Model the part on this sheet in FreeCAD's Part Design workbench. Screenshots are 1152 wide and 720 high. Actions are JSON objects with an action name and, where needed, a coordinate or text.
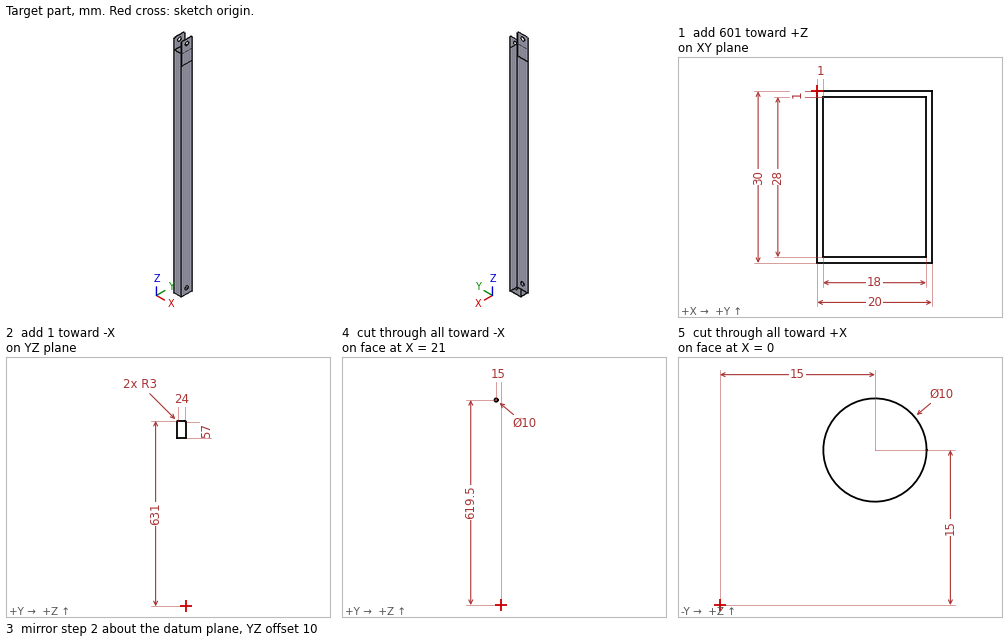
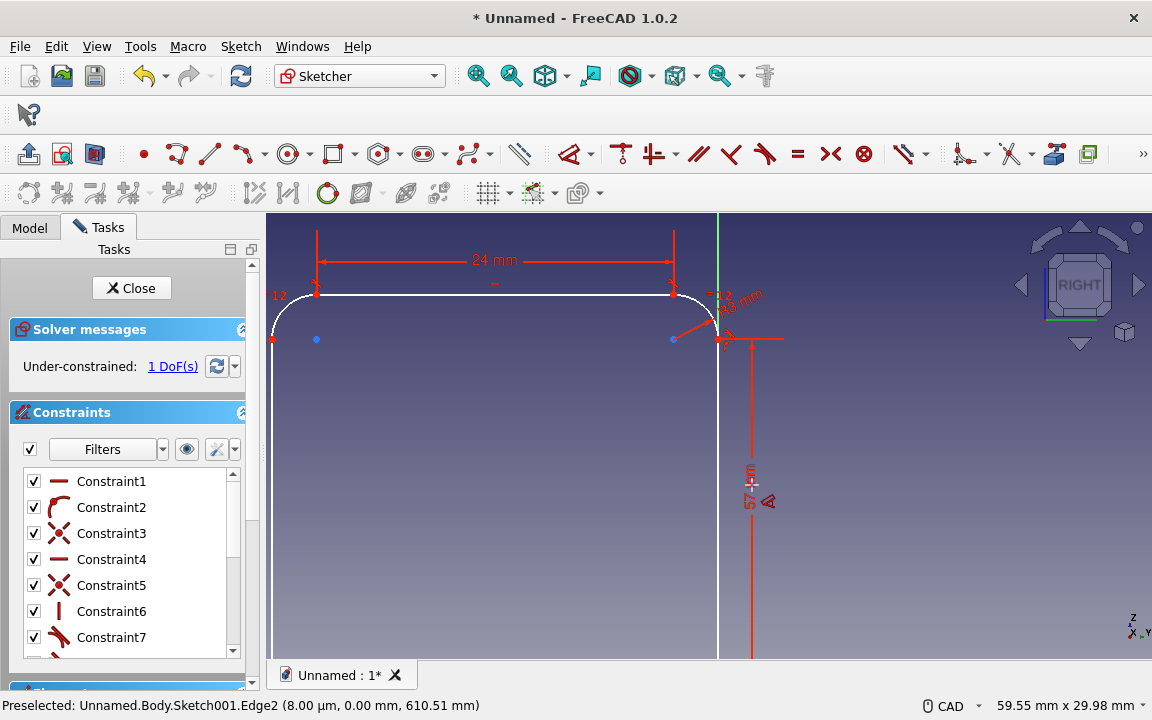
{"action": "left_click", "coordinate": [317, 295]}
{"action": "left_click", "coordinate": [752, 463]}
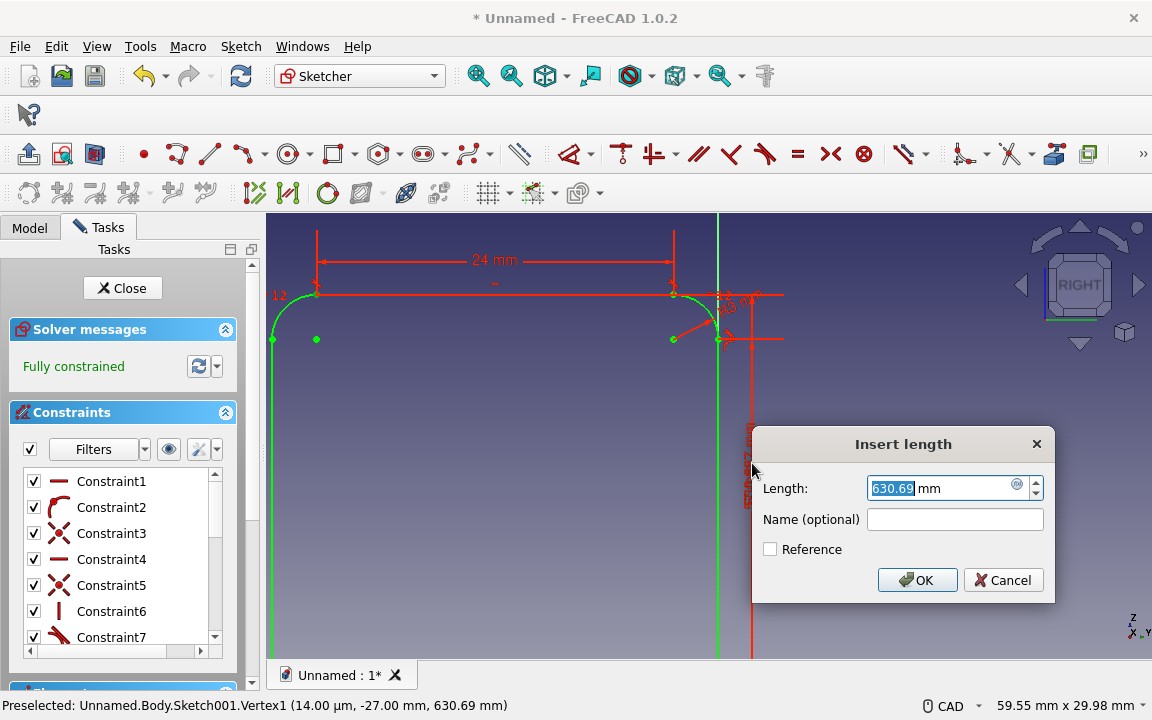
{"action": "type", "text": "631"}
{"action": "key", "text": "Return"}
{"action": "key", "text": "Escape"}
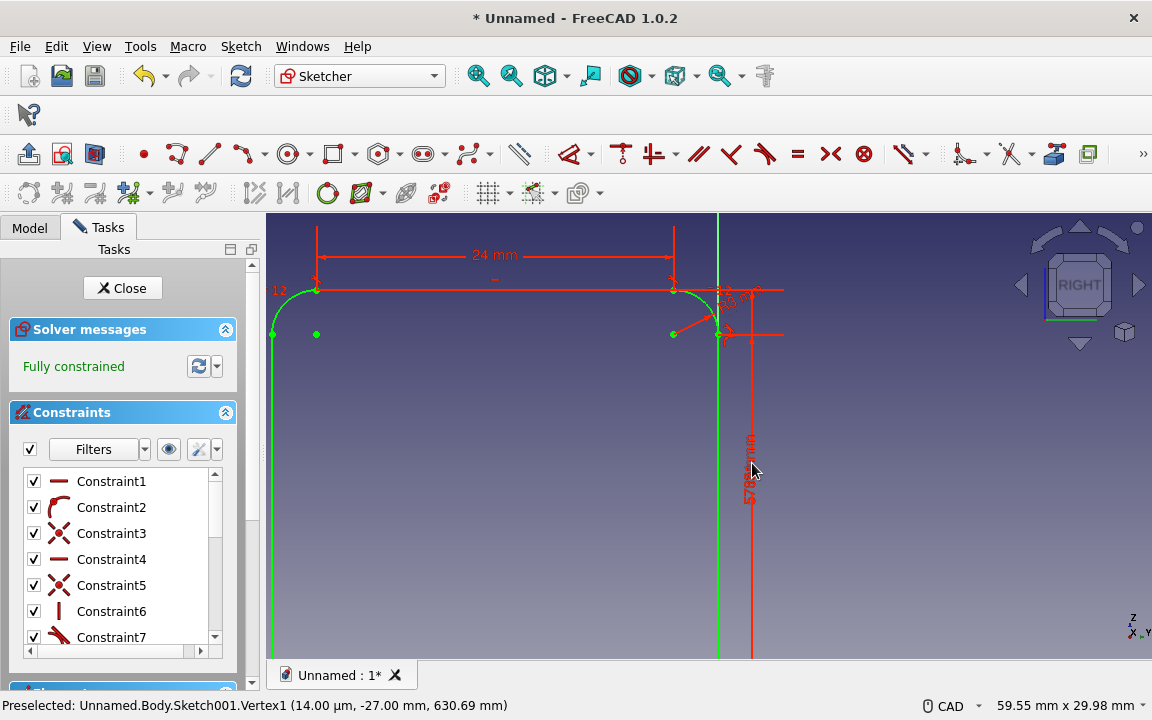
{"action": "left_click", "coordinate": [123, 288]}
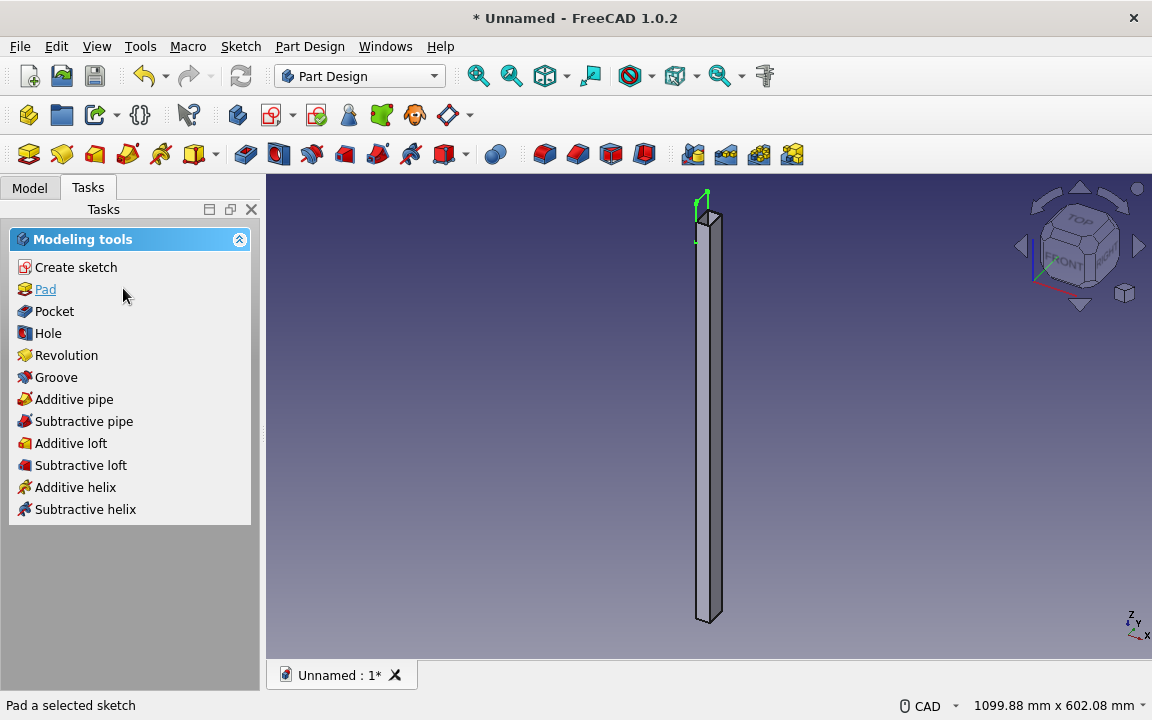
{"action": "left_click", "coordinate": [29, 154]}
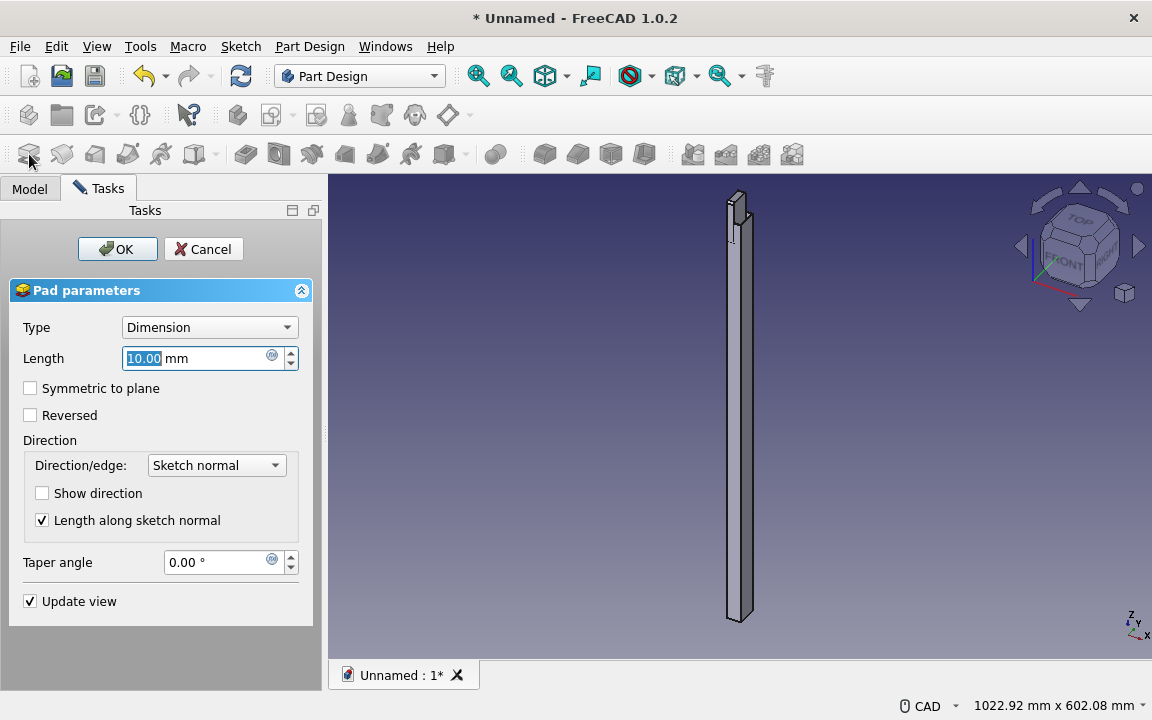
{"action": "type", "text": "1"}
{"action": "key", "text": "Tab"}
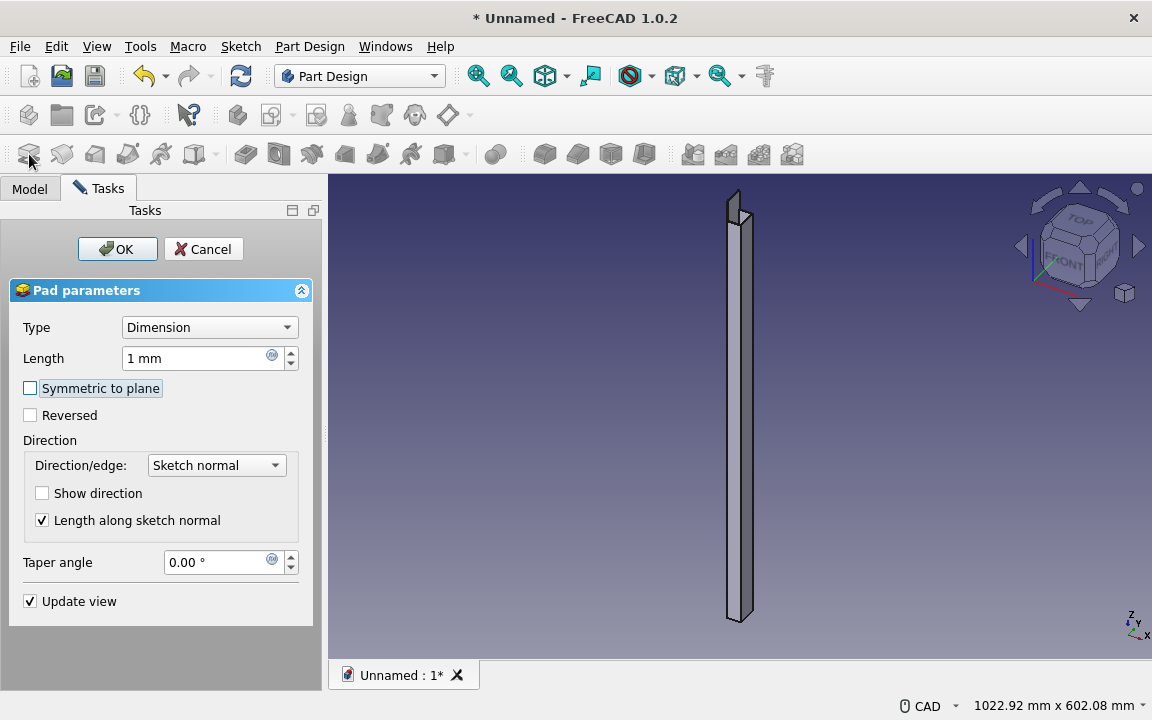
{"action": "left_click", "coordinate": [31, 415]}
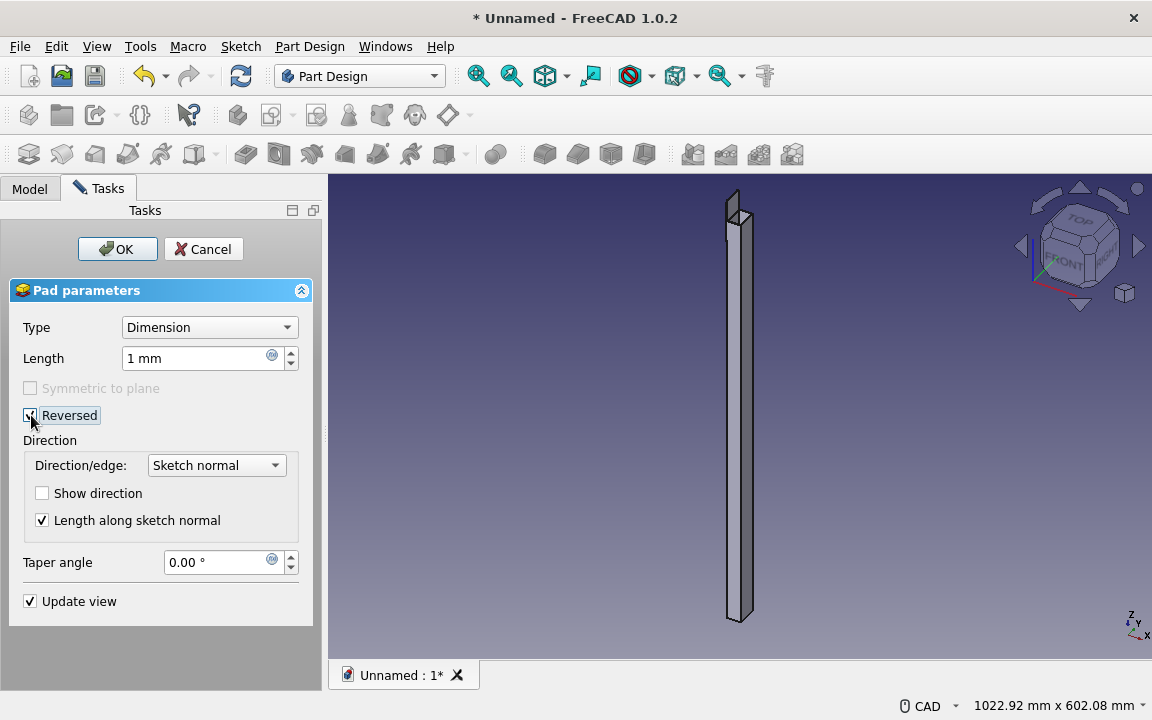
{"action": "left_click", "coordinate": [118, 249]}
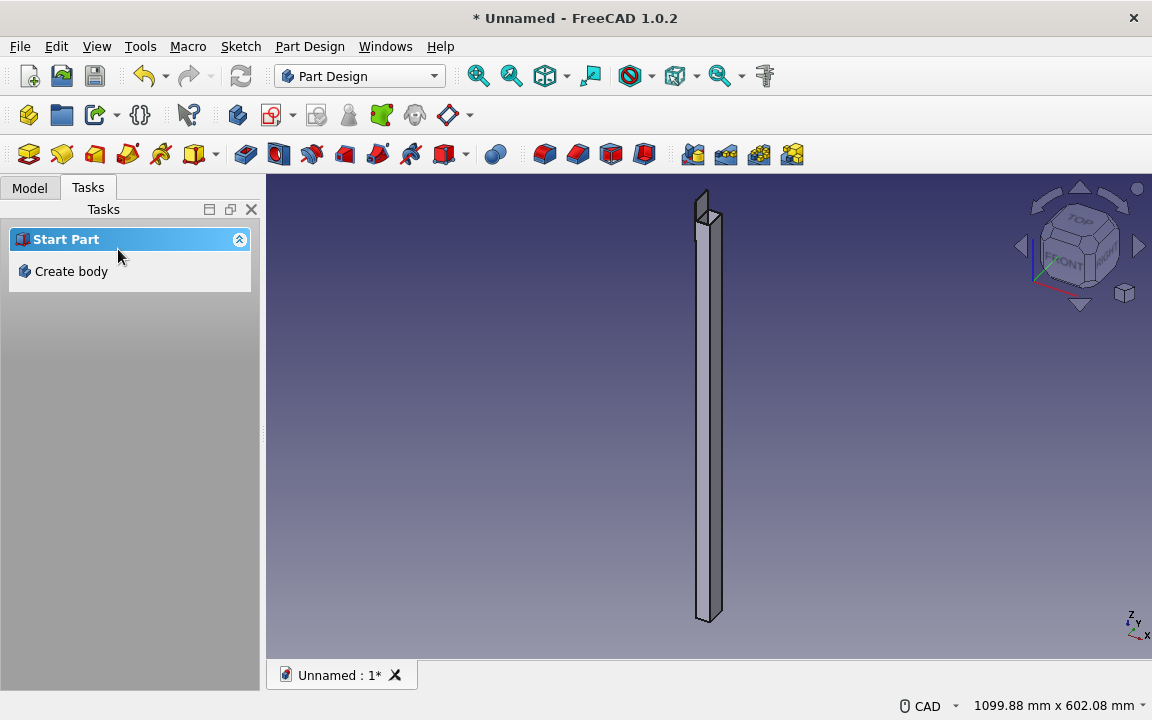
{"action": "left_click", "coordinate": [30, 188]}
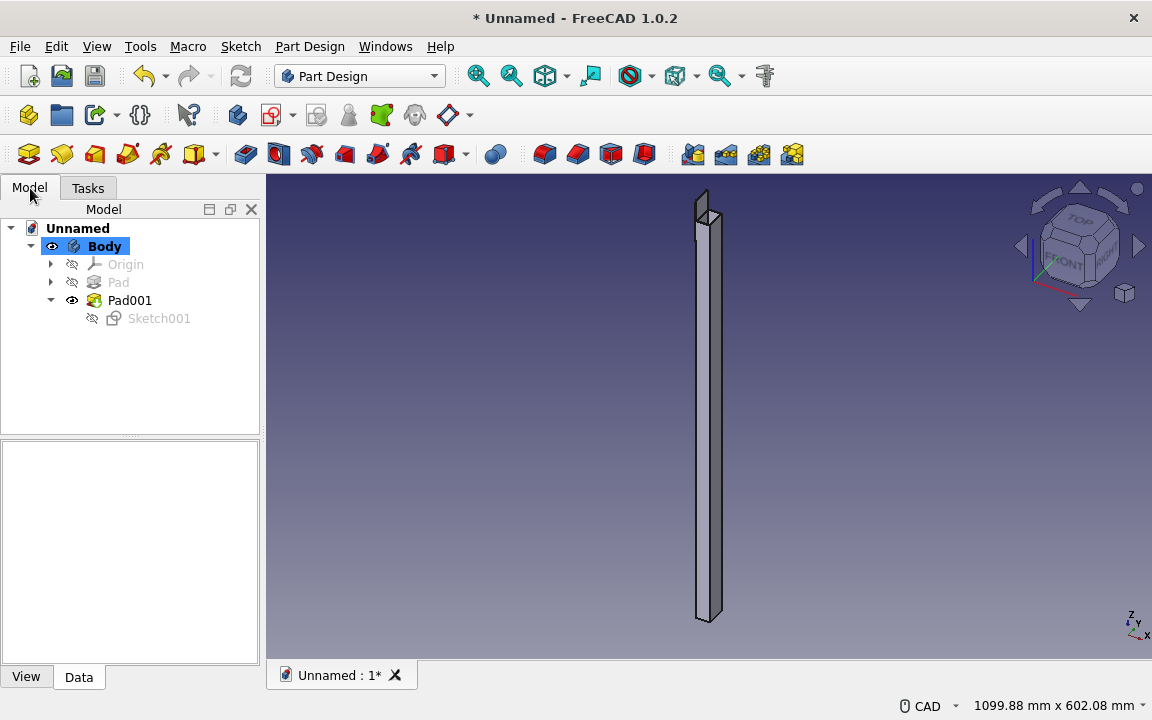
{"action": "left_click", "coordinate": [51, 264]}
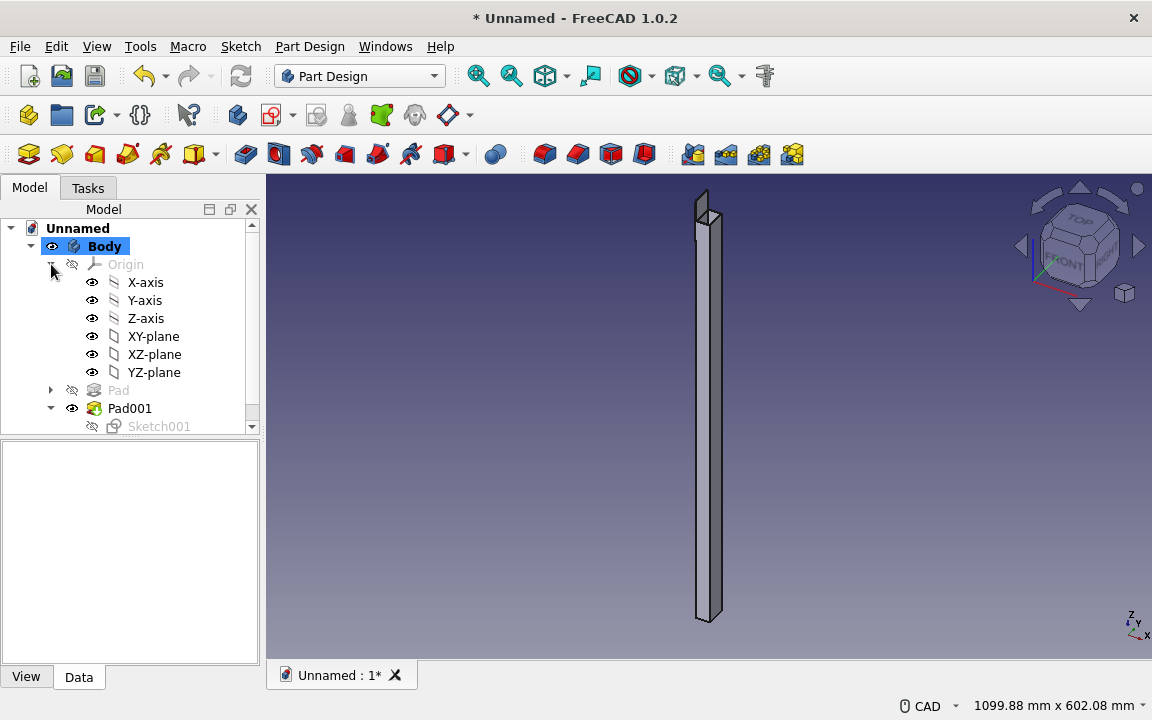
{"action": "left_click", "coordinate": [137, 372]}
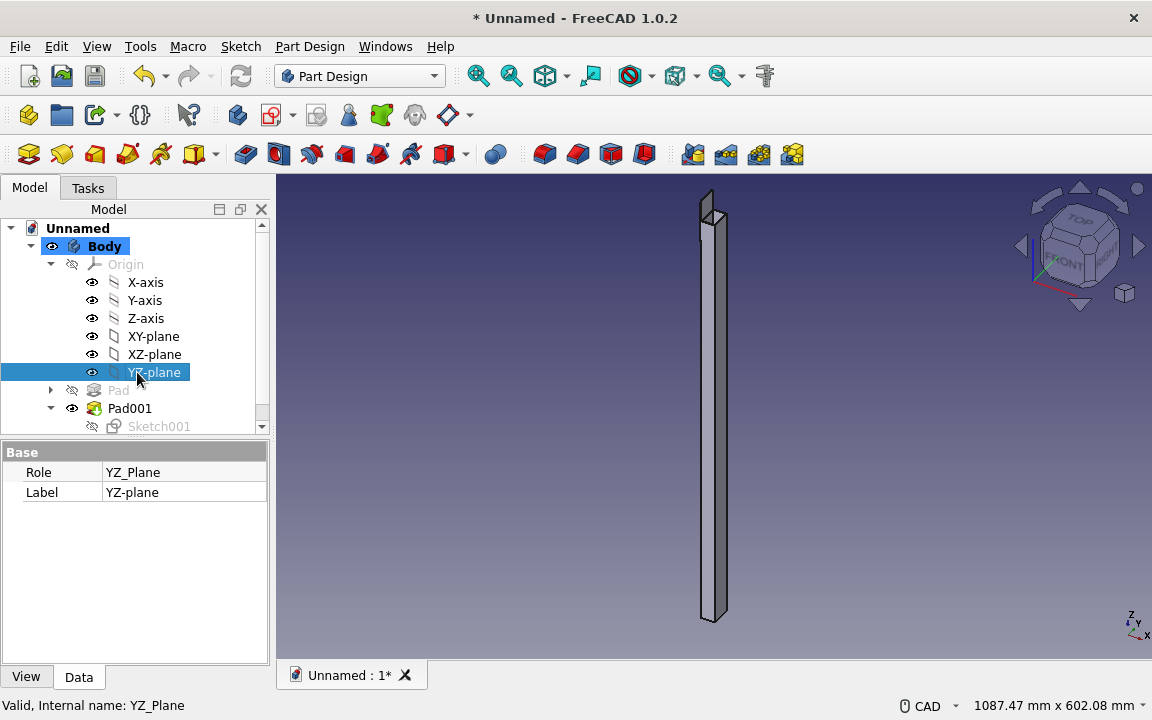
{"action": "left_click", "coordinate": [448, 116]}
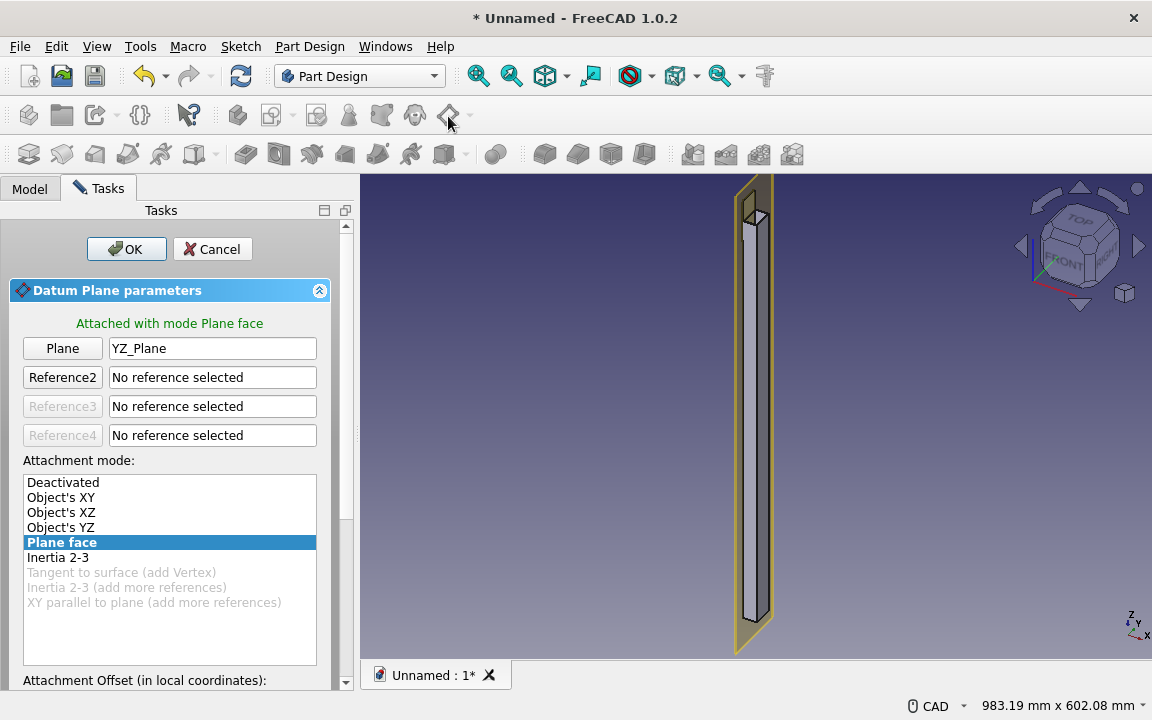
{"action": "scroll", "coordinate": [346, 455], "scroll_direction": "down", "scroll_amount": 3}